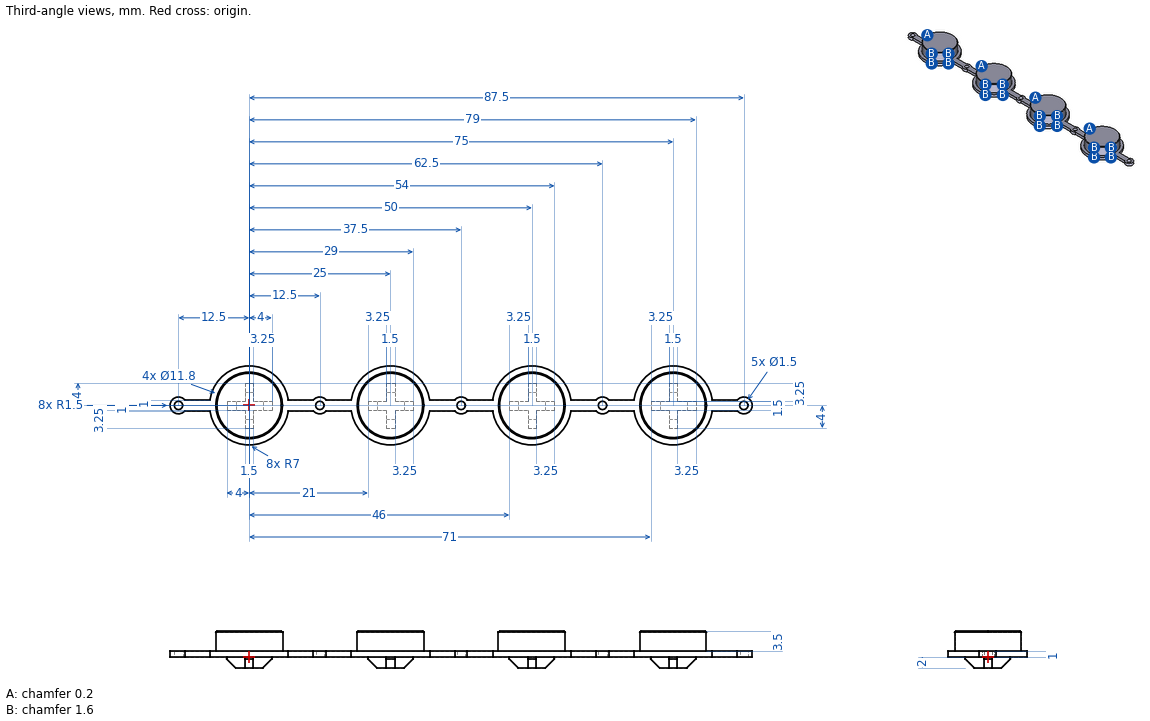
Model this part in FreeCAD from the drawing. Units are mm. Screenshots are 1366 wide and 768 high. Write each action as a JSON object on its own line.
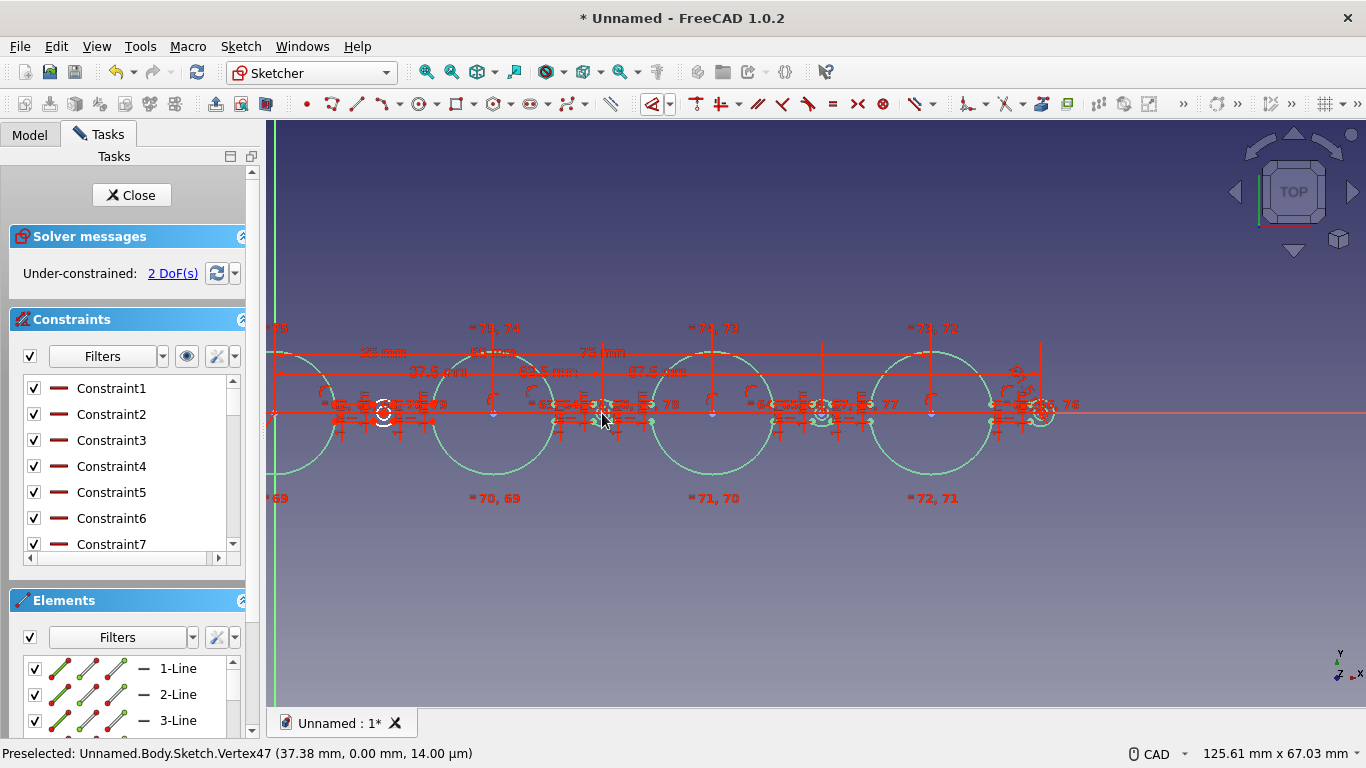
{"action": "left_click", "coordinate": [384, 413]}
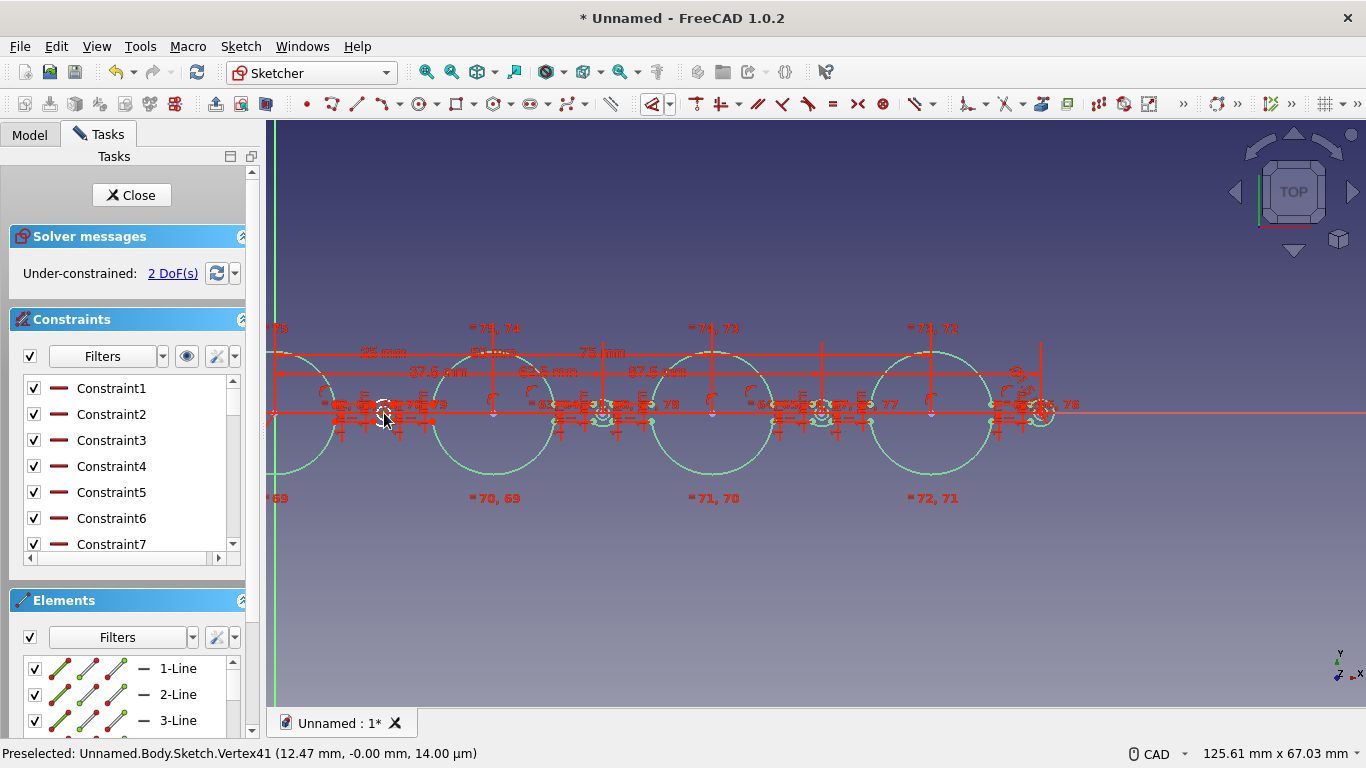
{"action": "key", "text": "l"}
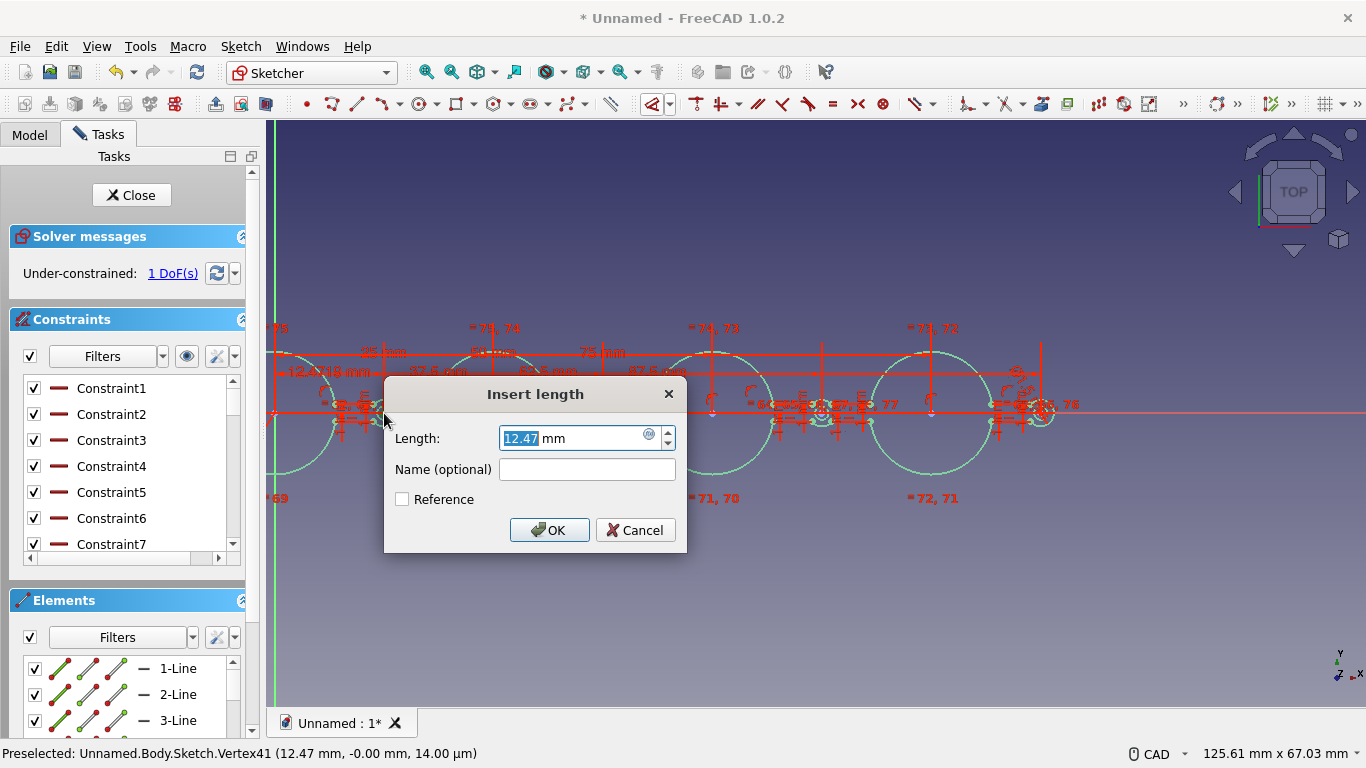
{"action": "type", "text": "12.5"}
{"action": "key", "text": "Return"}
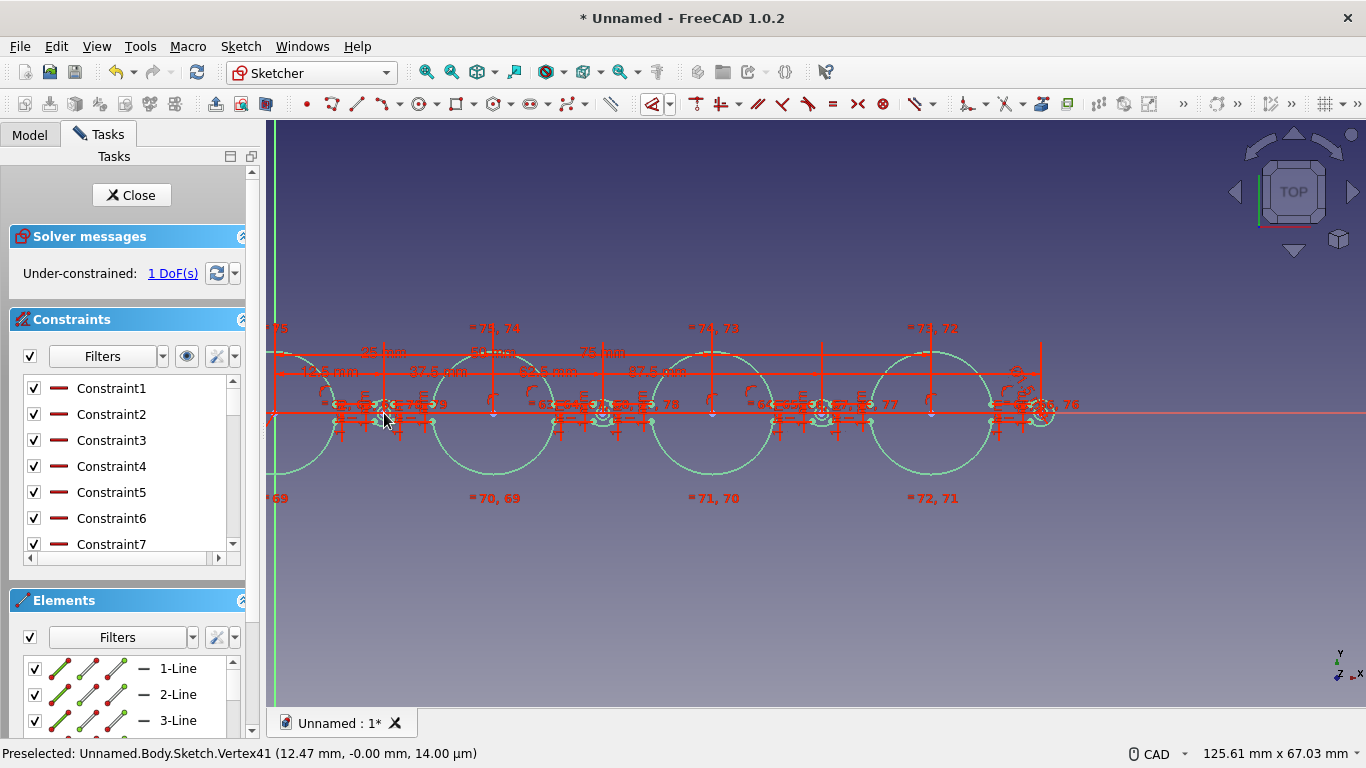
{"action": "scroll", "coordinate": [1041, 414], "scroll_direction": "down", "scroll_amount": 2}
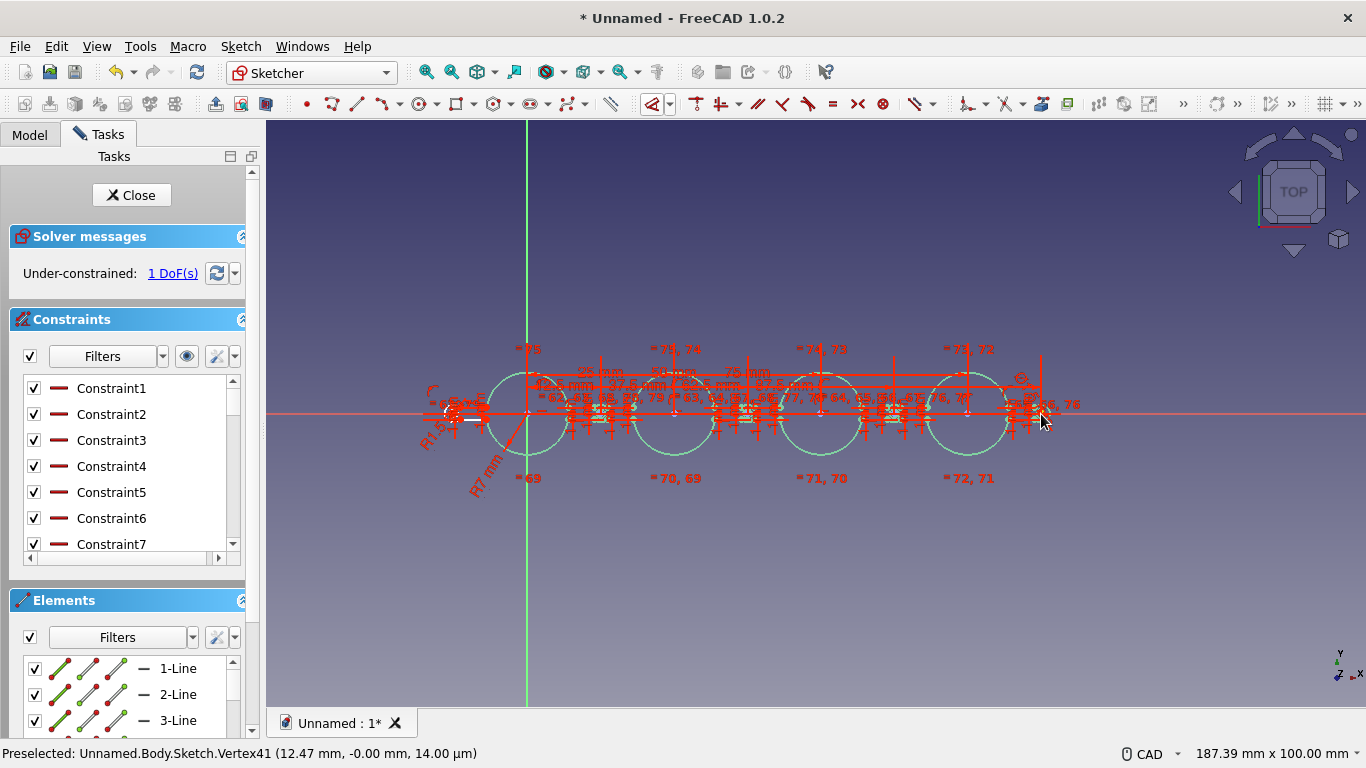
{"action": "scroll", "coordinate": [453, 414], "scroll_direction": "up", "scroll_amount": 2}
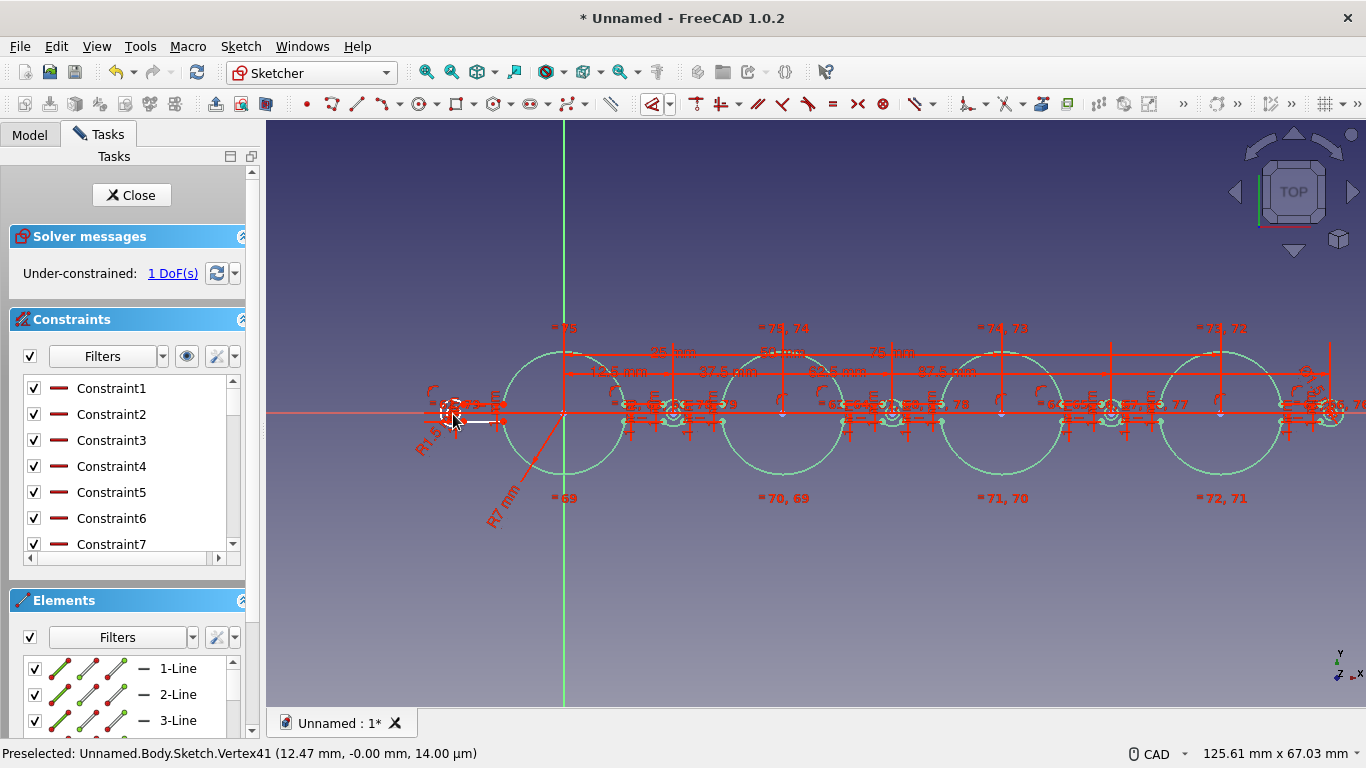
{"action": "left_click", "coordinate": [454, 413]}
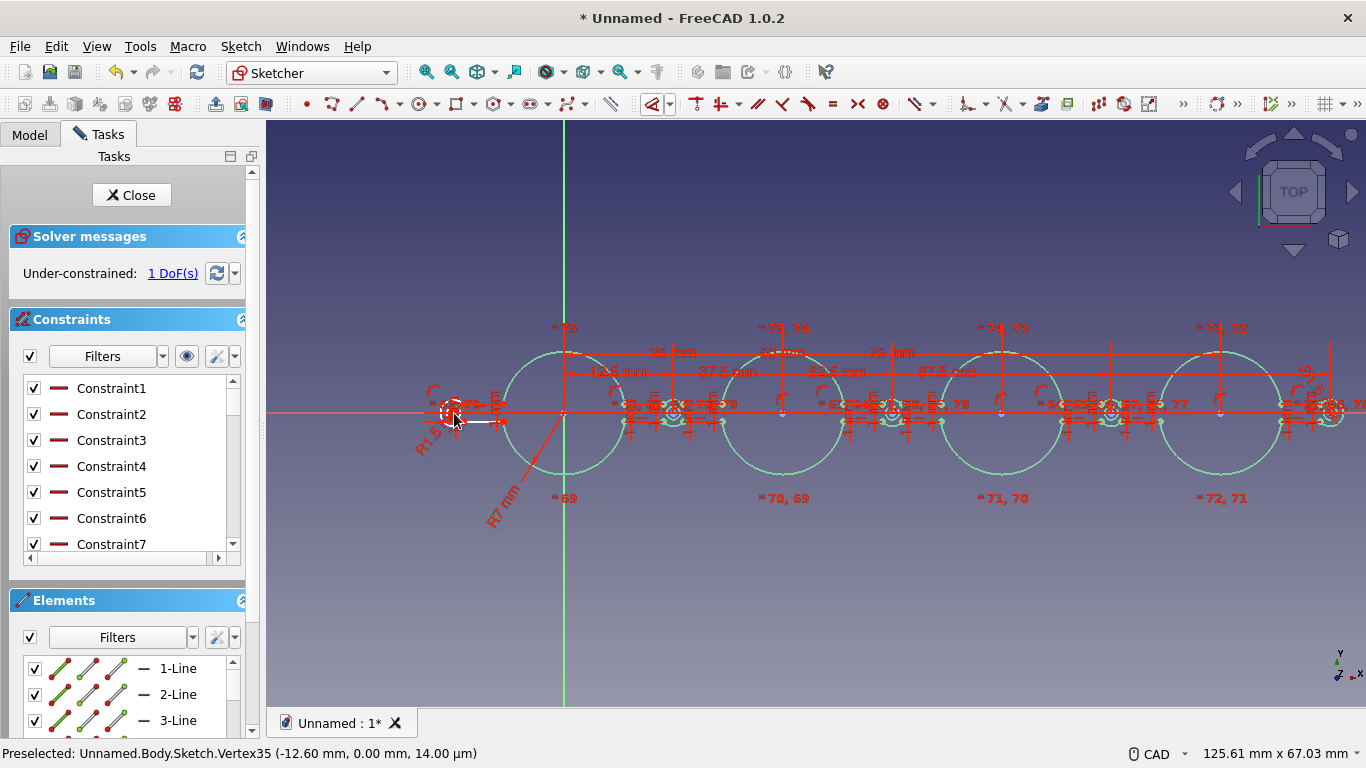
{"action": "left_click", "coordinate": [670, 104]}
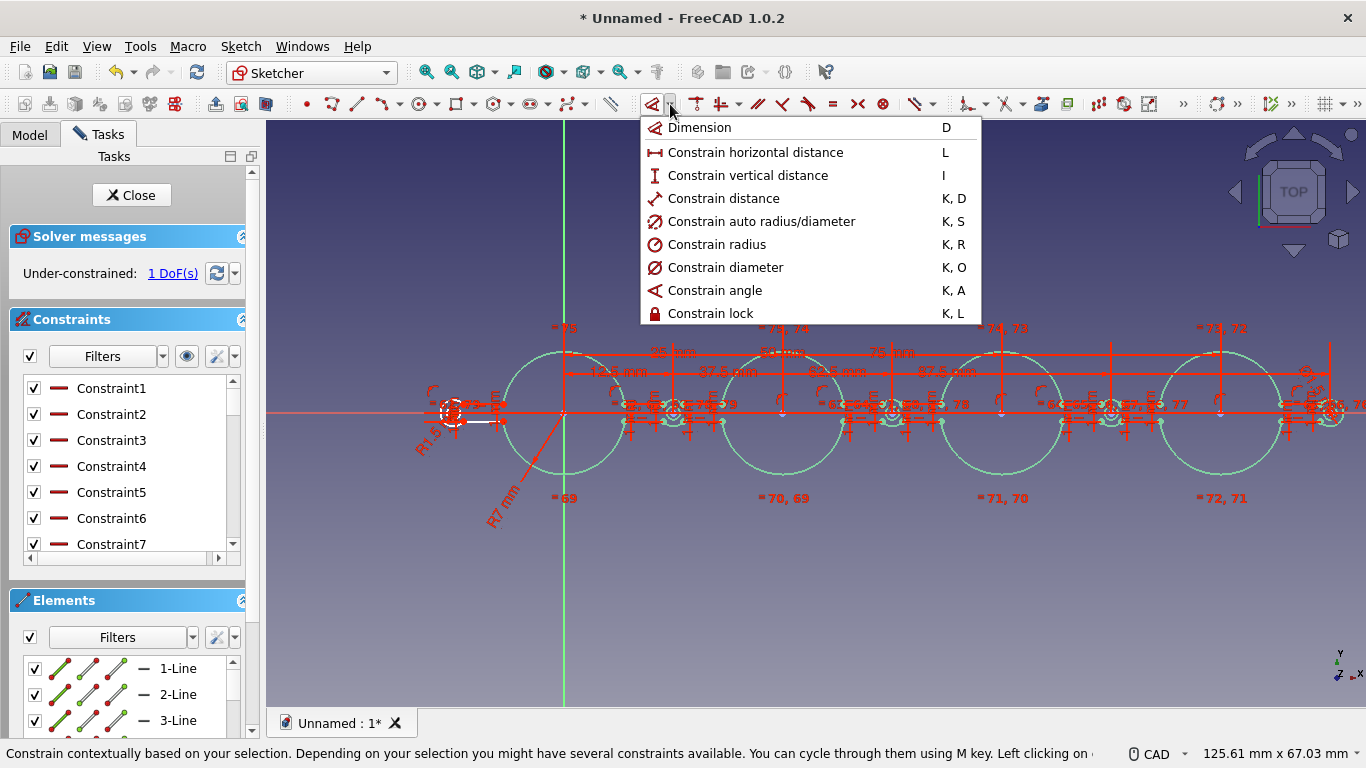
{"action": "left_click", "coordinate": [811, 152]}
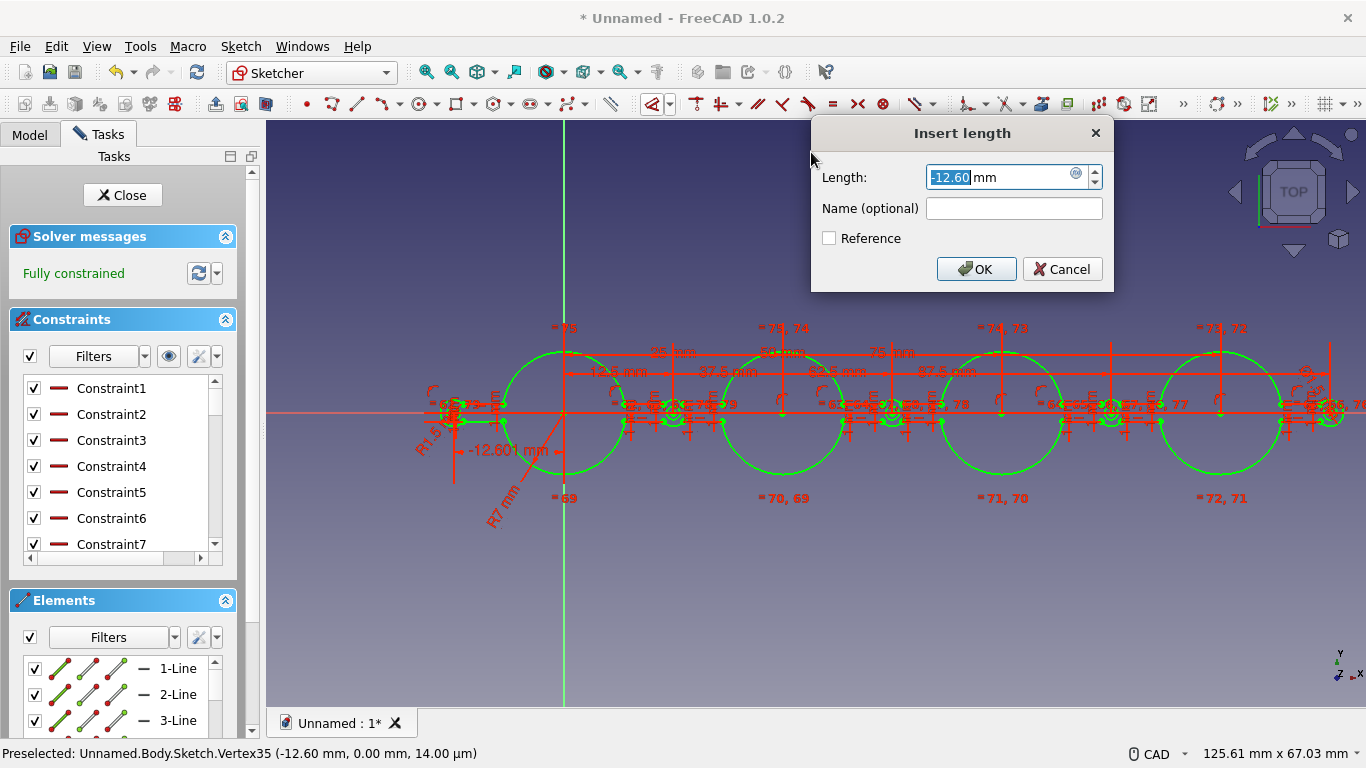
{"action": "type", "text": "-12.5"}
{"action": "key", "text": "Return"}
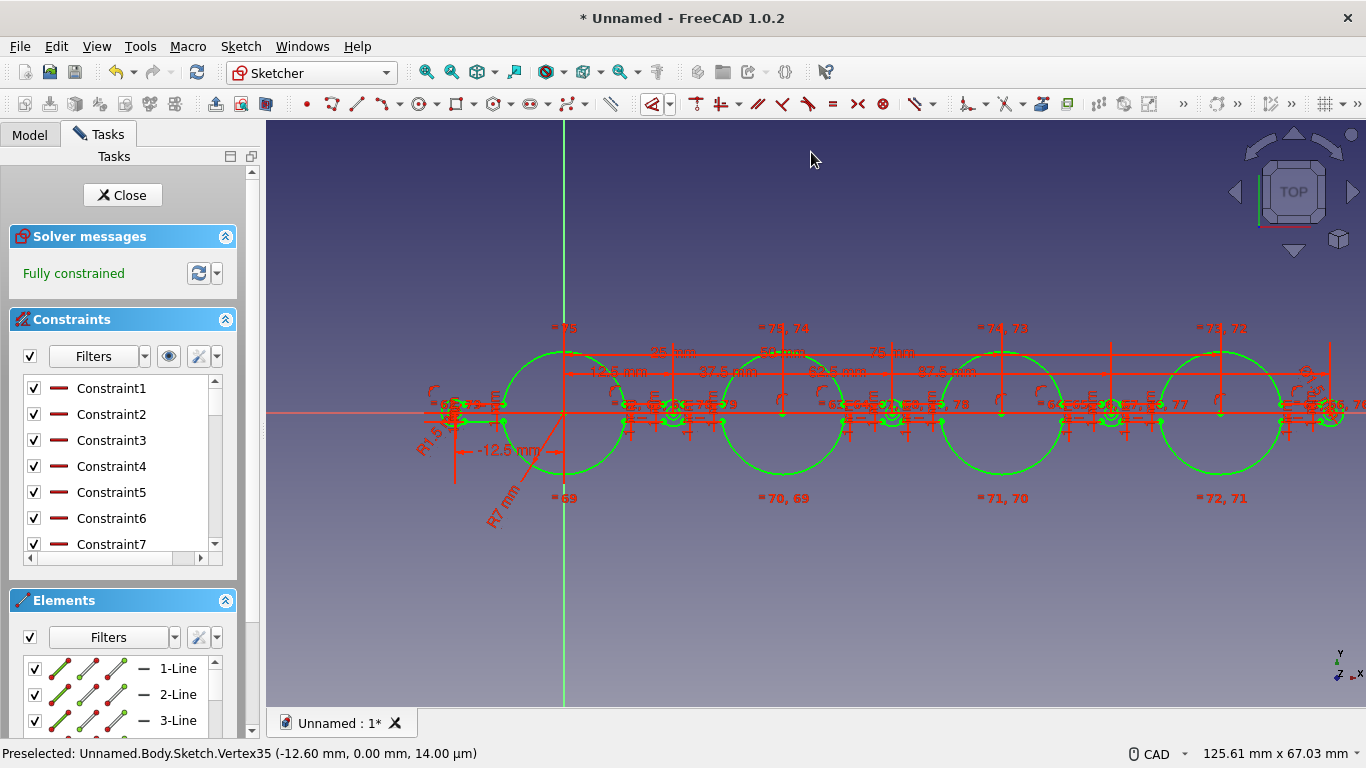
{"action": "left_click", "coordinate": [123, 195]}